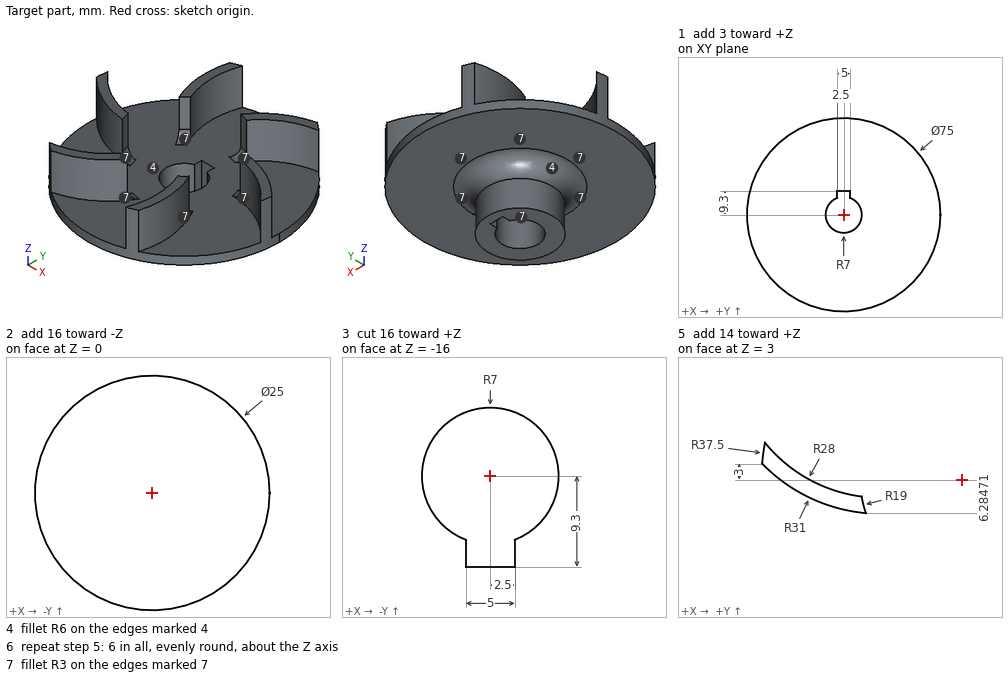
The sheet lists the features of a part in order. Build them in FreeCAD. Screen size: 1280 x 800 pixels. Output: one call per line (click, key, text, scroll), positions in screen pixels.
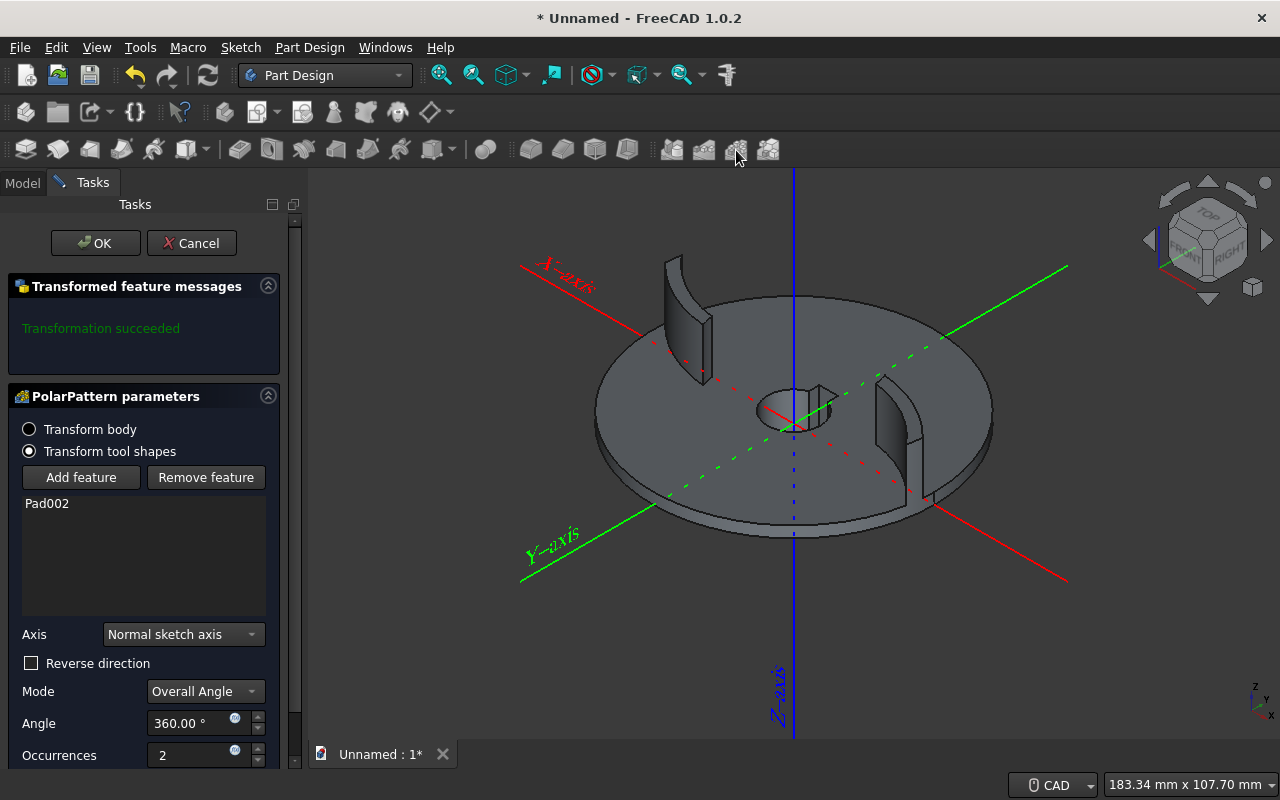
click(184, 634)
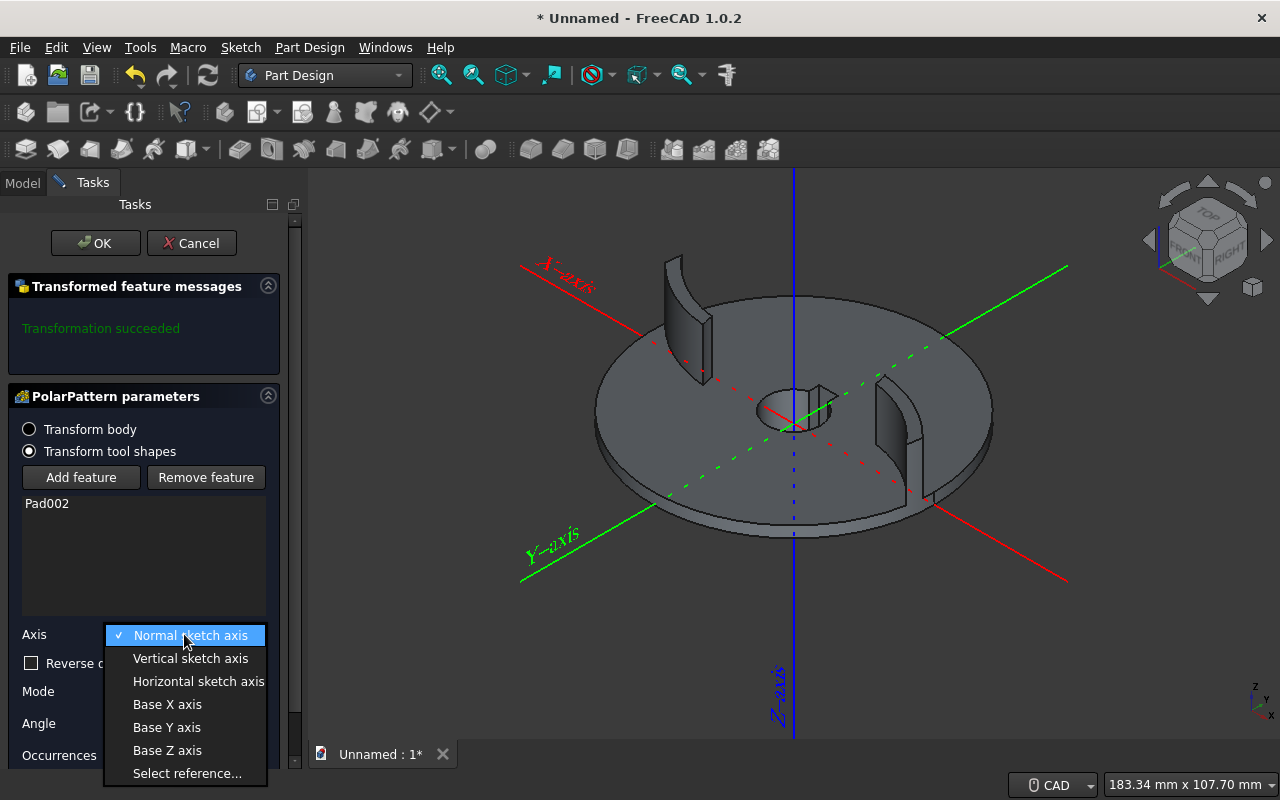
click(184, 750)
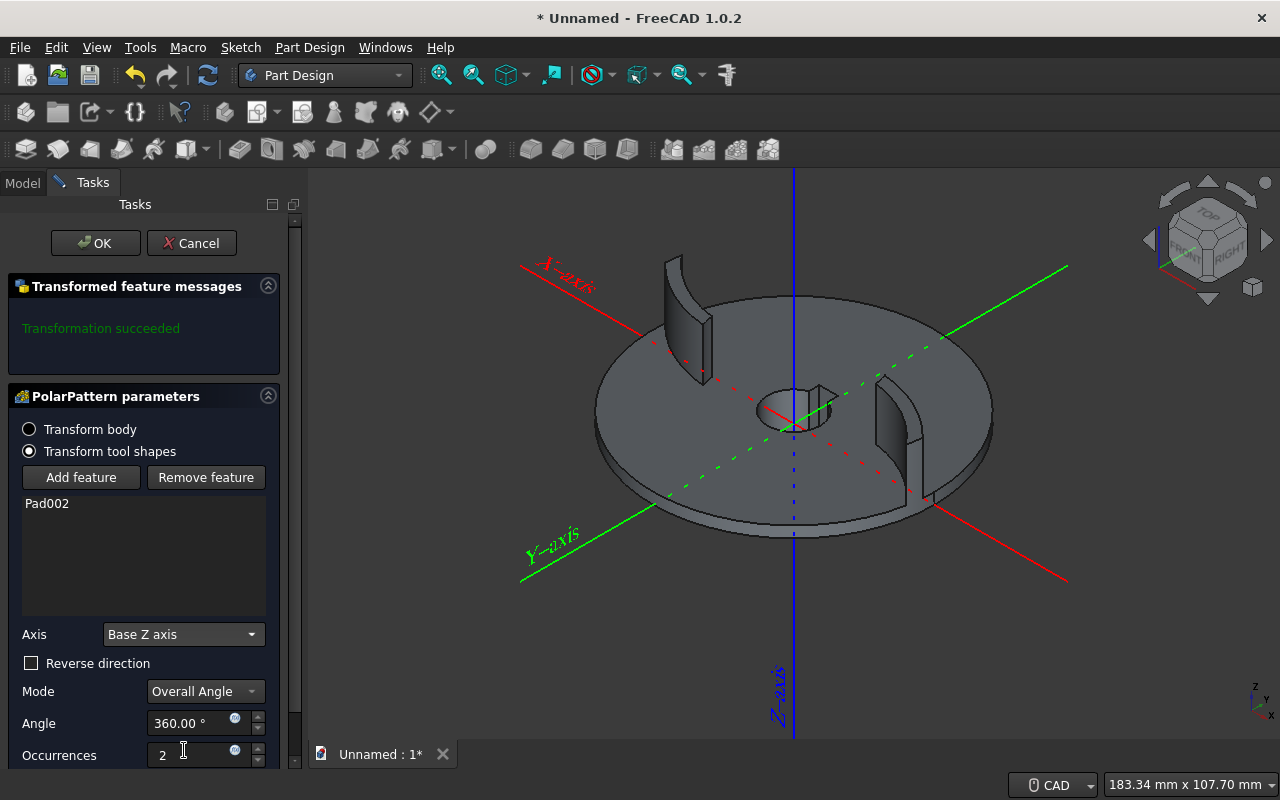
triple_click(198, 755)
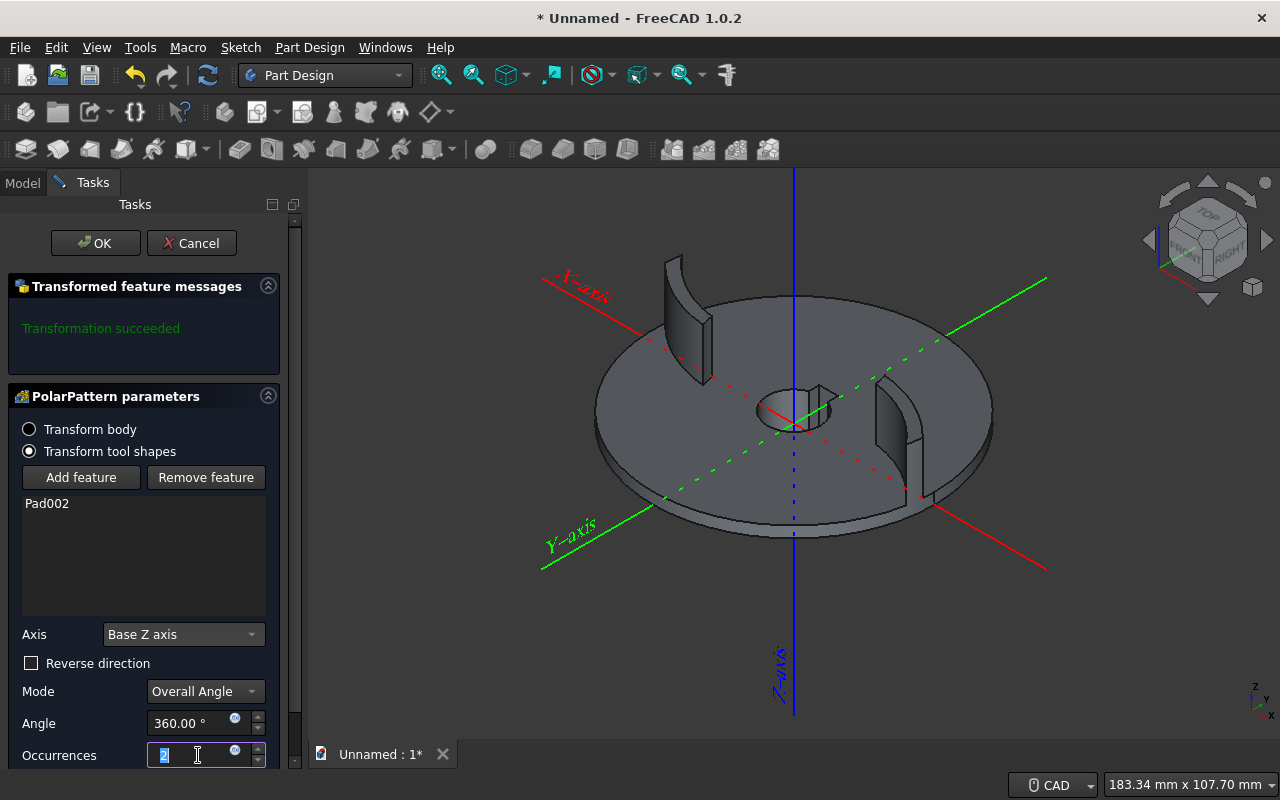
text(6)
key(Tab)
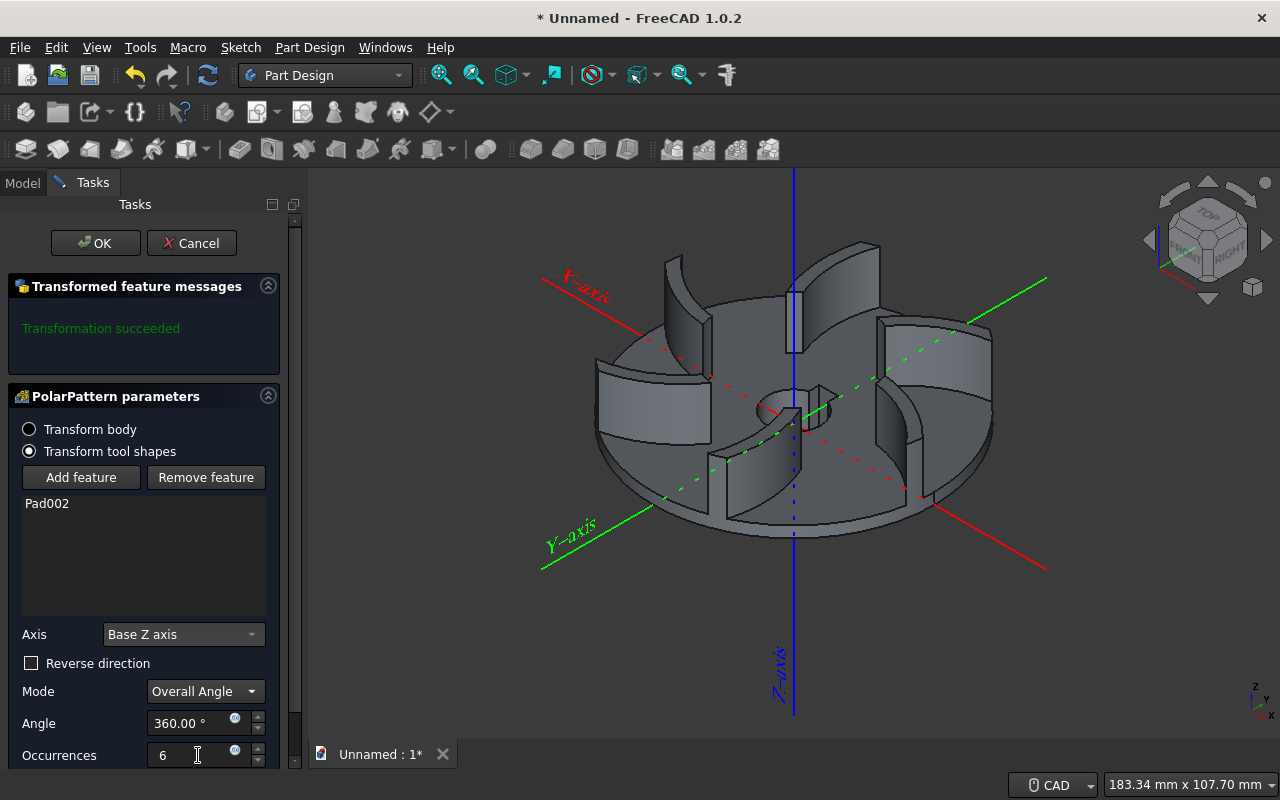
click(96, 243)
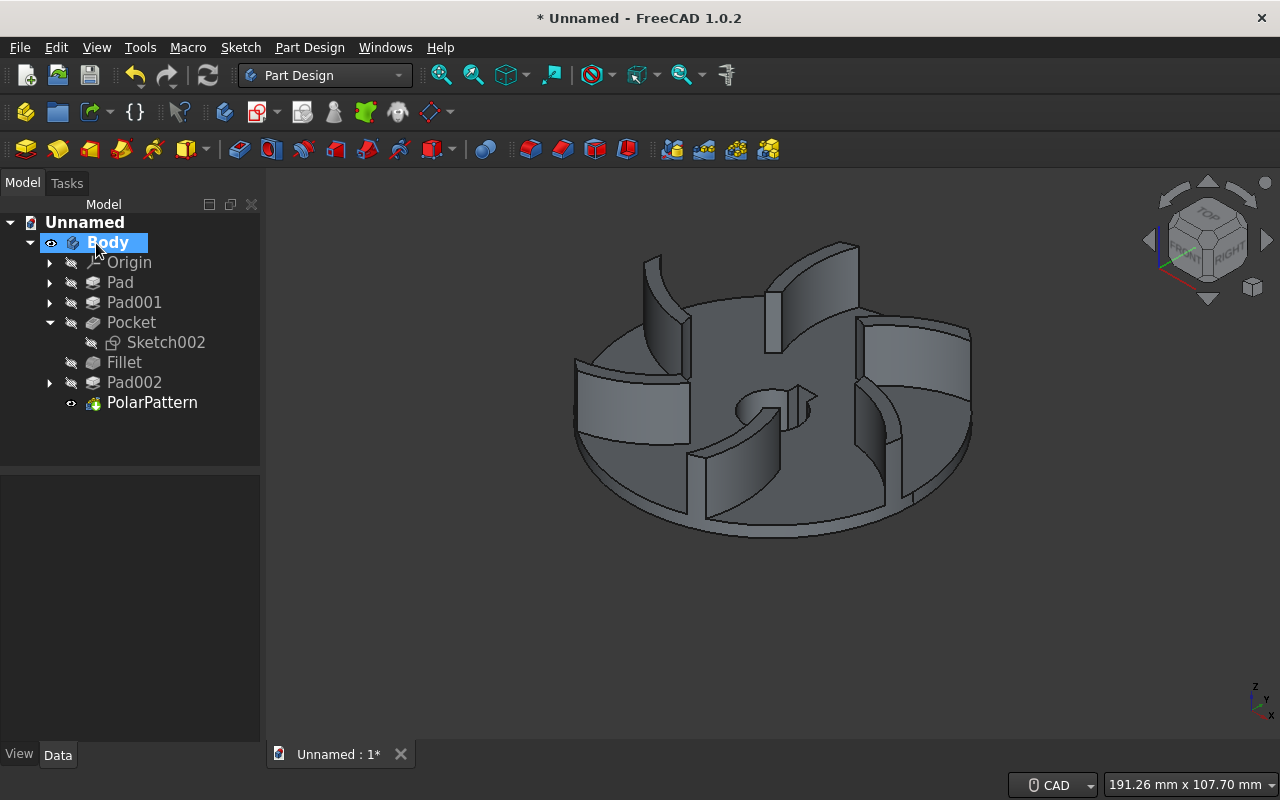
scroll(774, 352, up, 5)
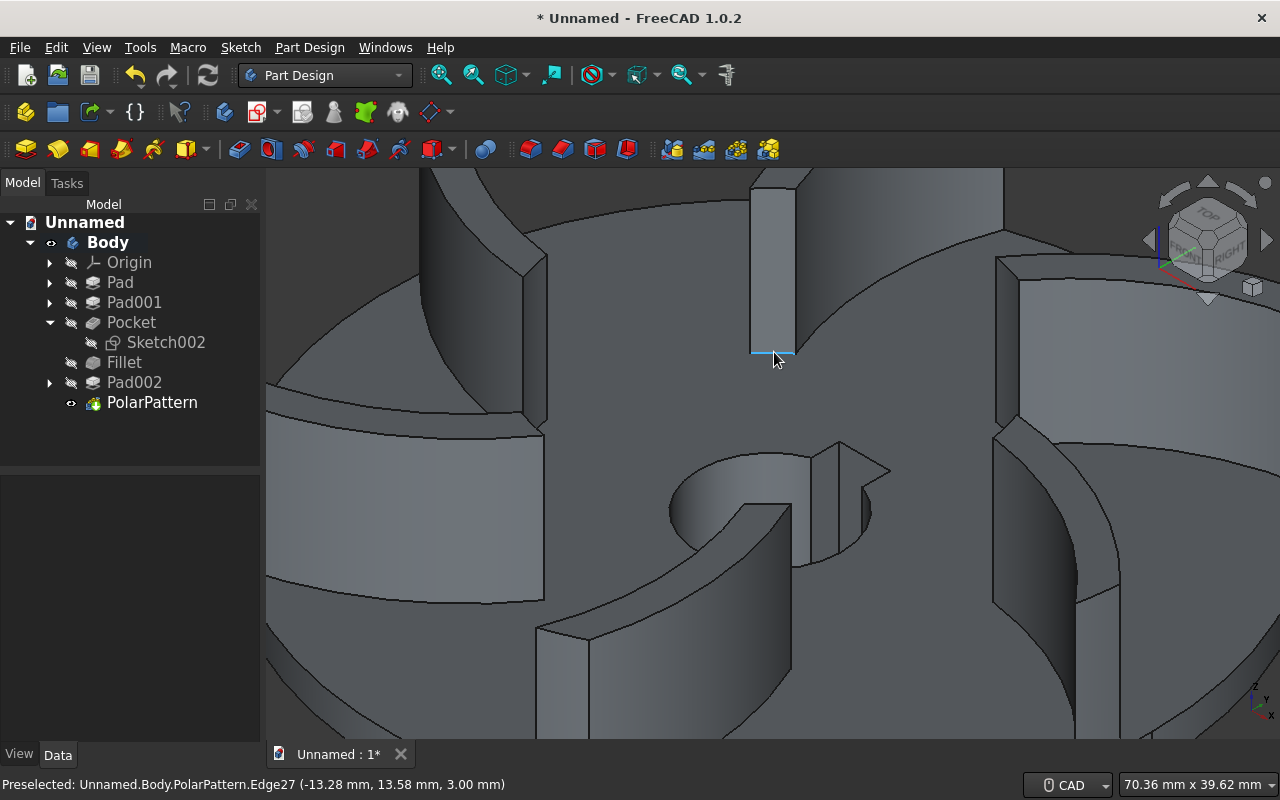
key(v)
key(f)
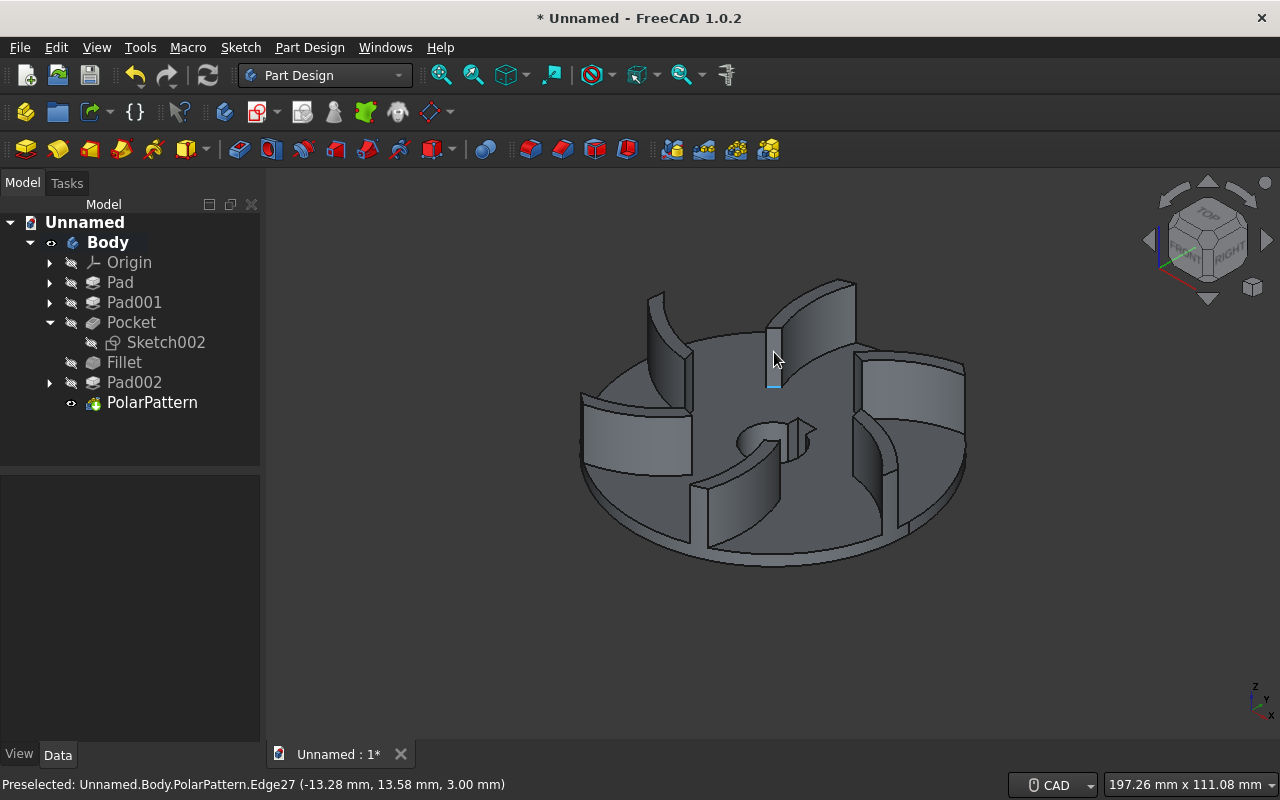
key(2)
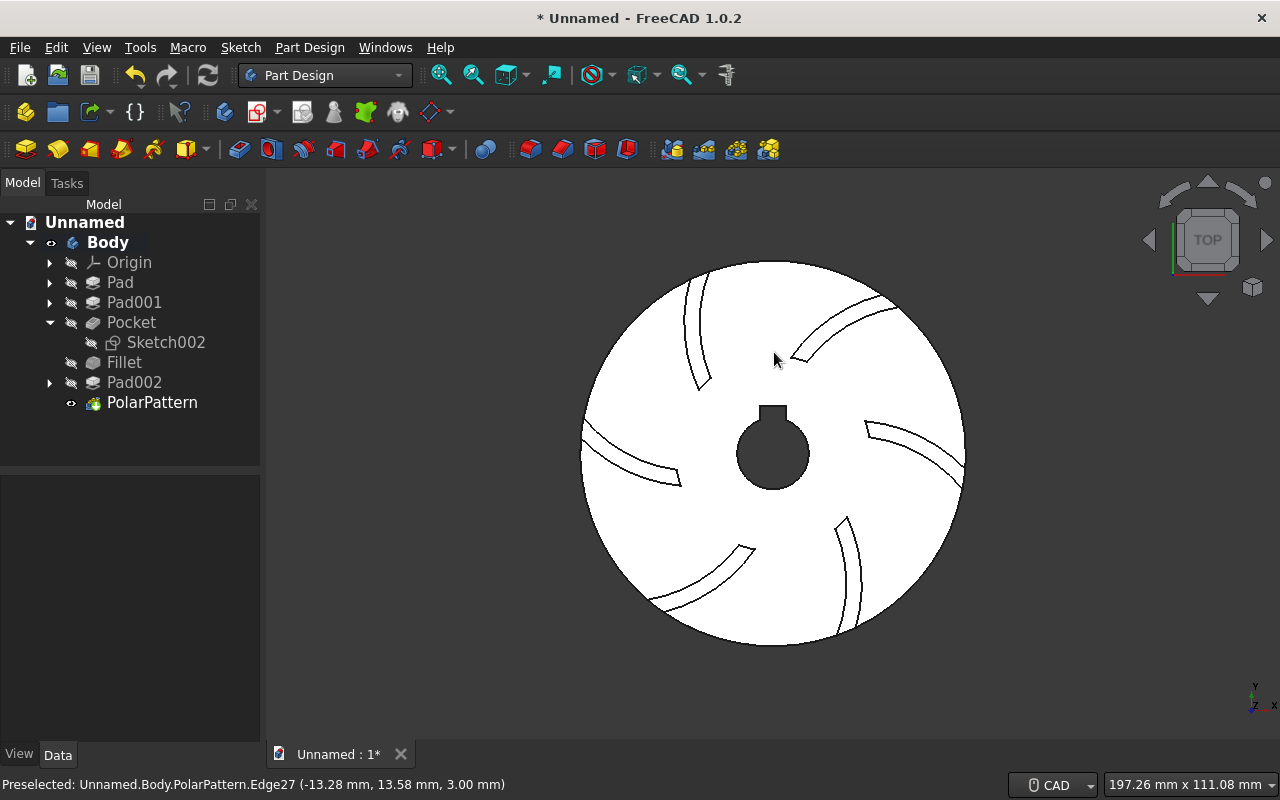
scroll(705, 383, up, 5)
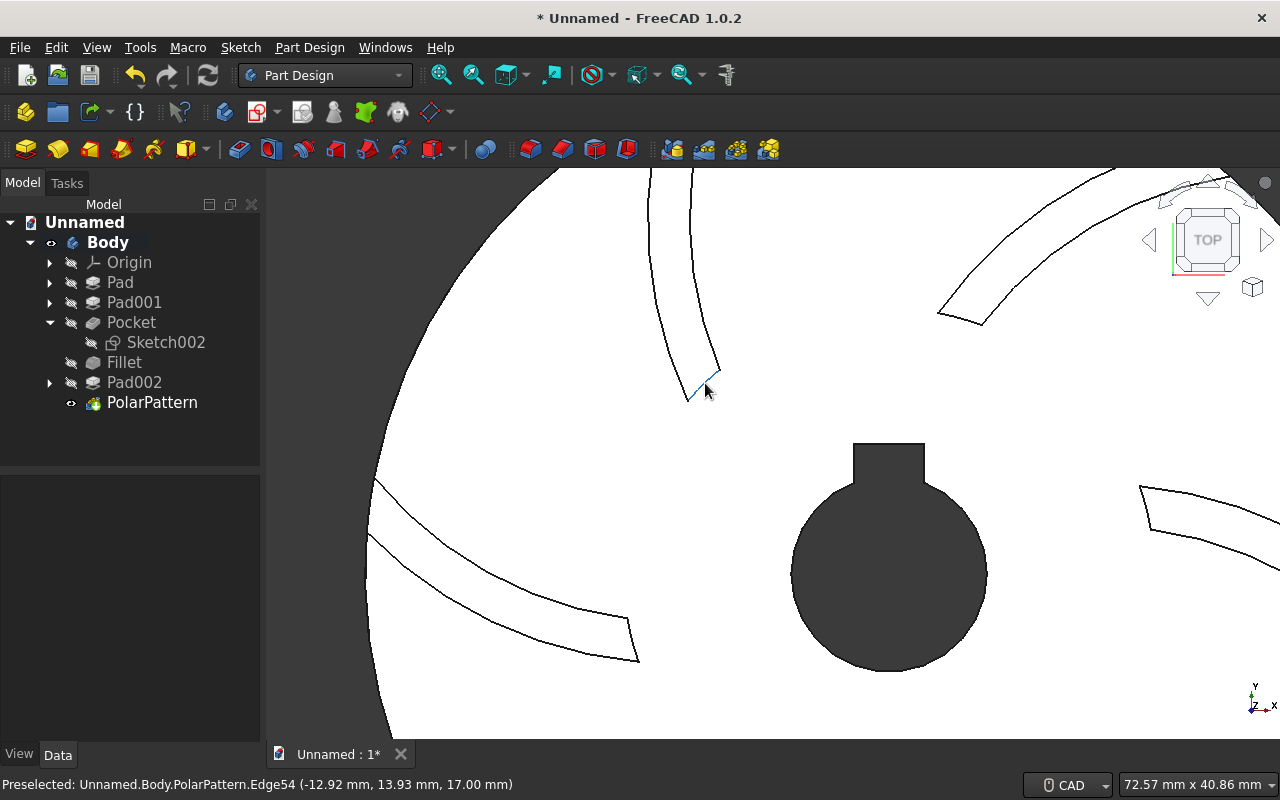
key(v)
key(f)